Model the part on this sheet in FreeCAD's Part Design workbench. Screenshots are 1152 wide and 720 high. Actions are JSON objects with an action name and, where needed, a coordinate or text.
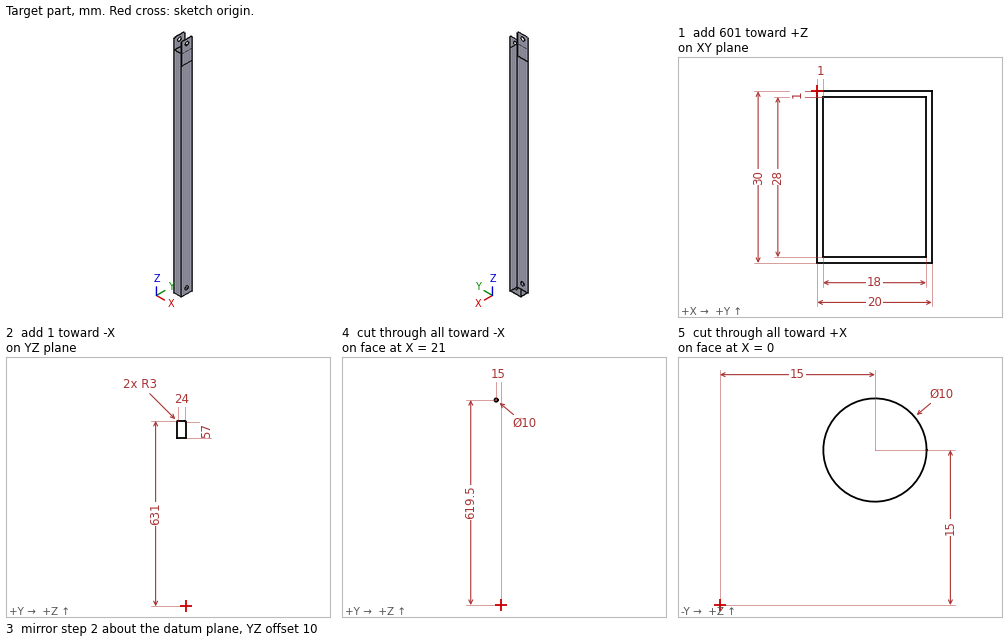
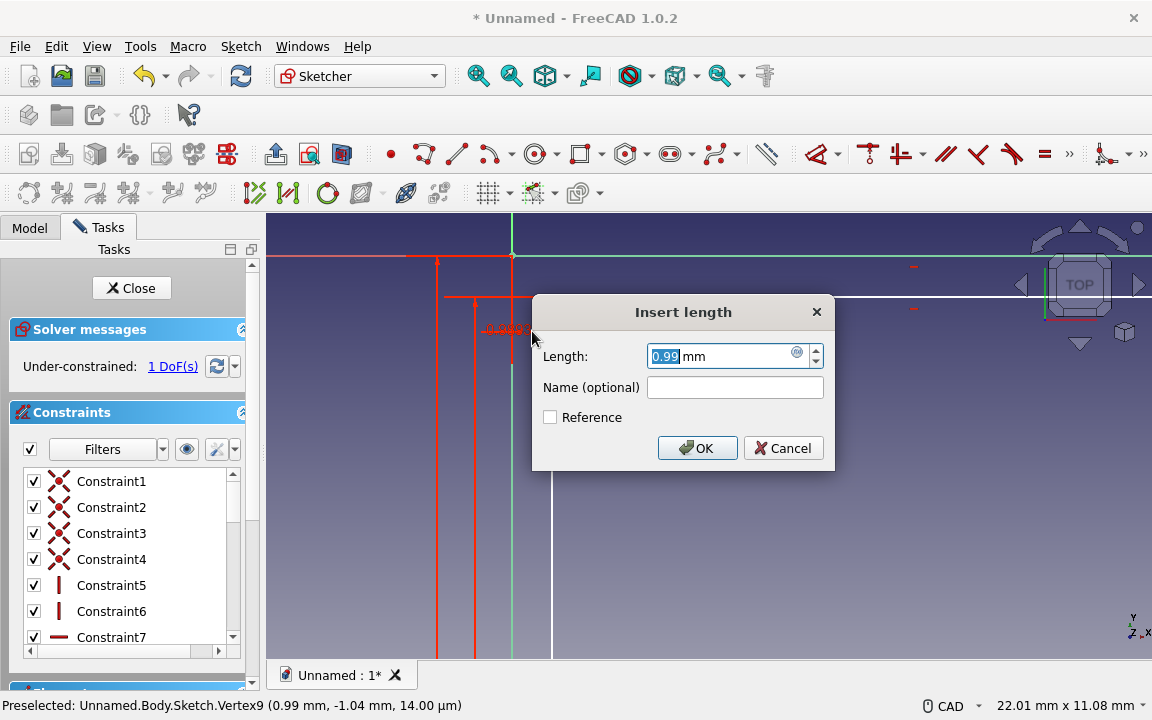
{"action": "type", "text": "1"}
{"action": "key", "text": "Return"}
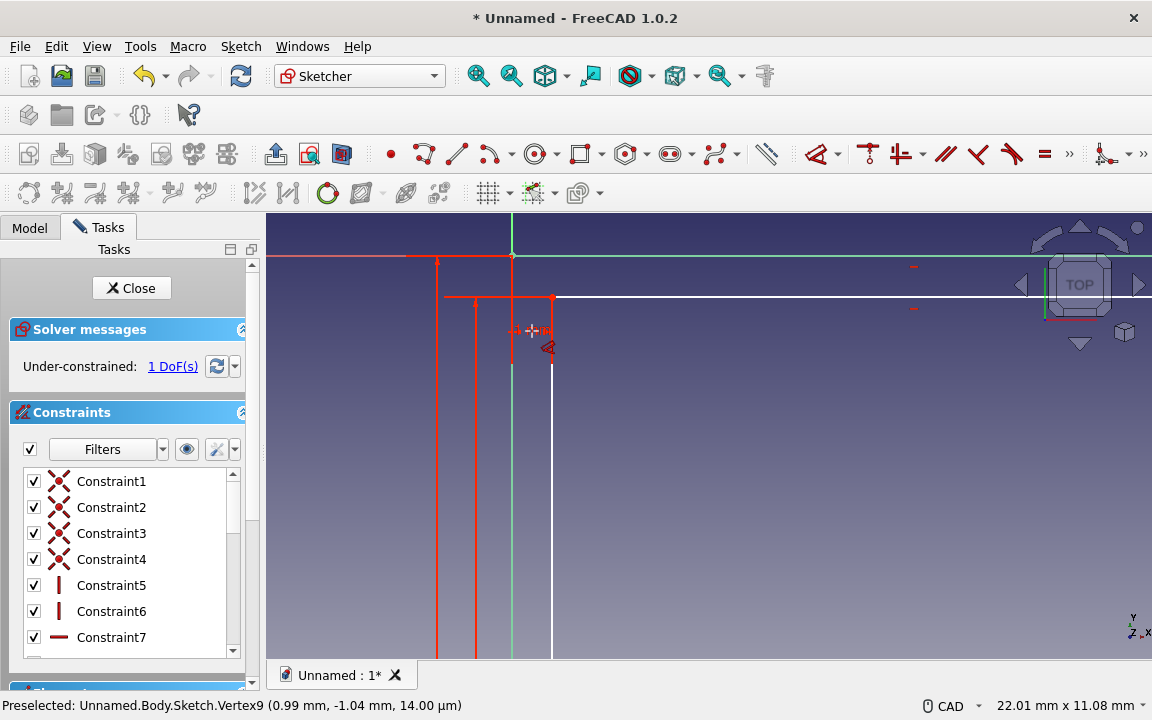
{"action": "left_click", "coordinate": [552, 297]}
{"action": "left_click", "coordinate": [478, 276]}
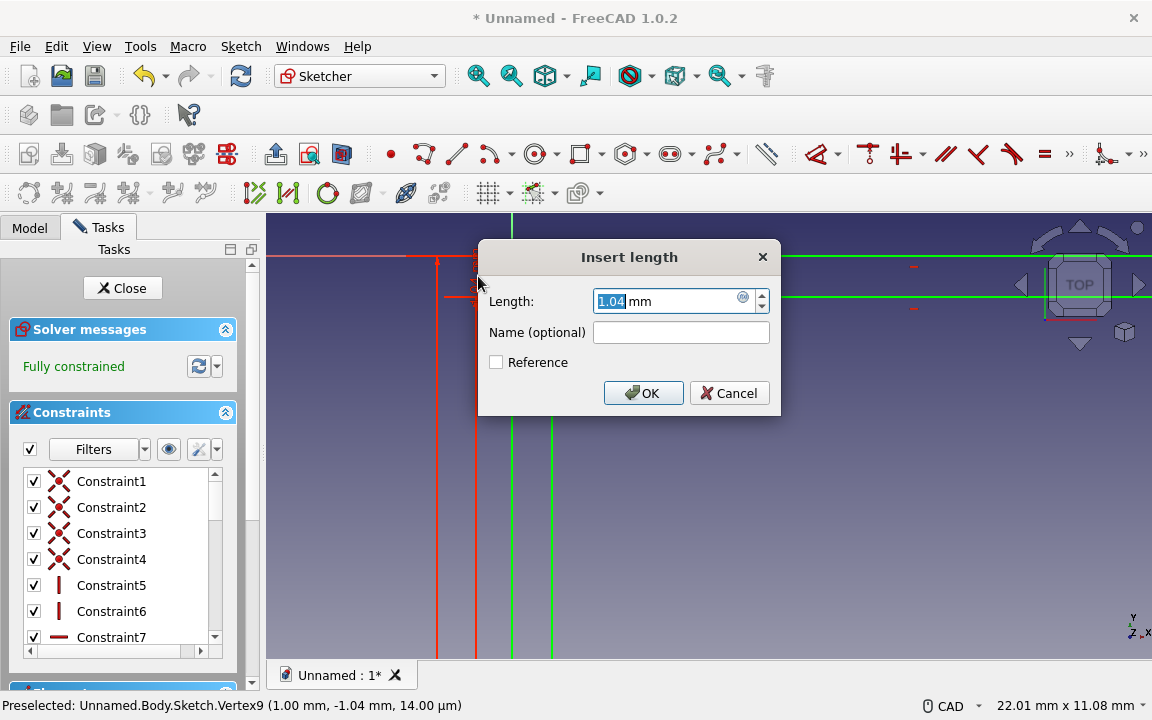
{"action": "type", "text": "1"}
{"action": "key", "text": "Return"}
{"action": "key", "text": "Escape"}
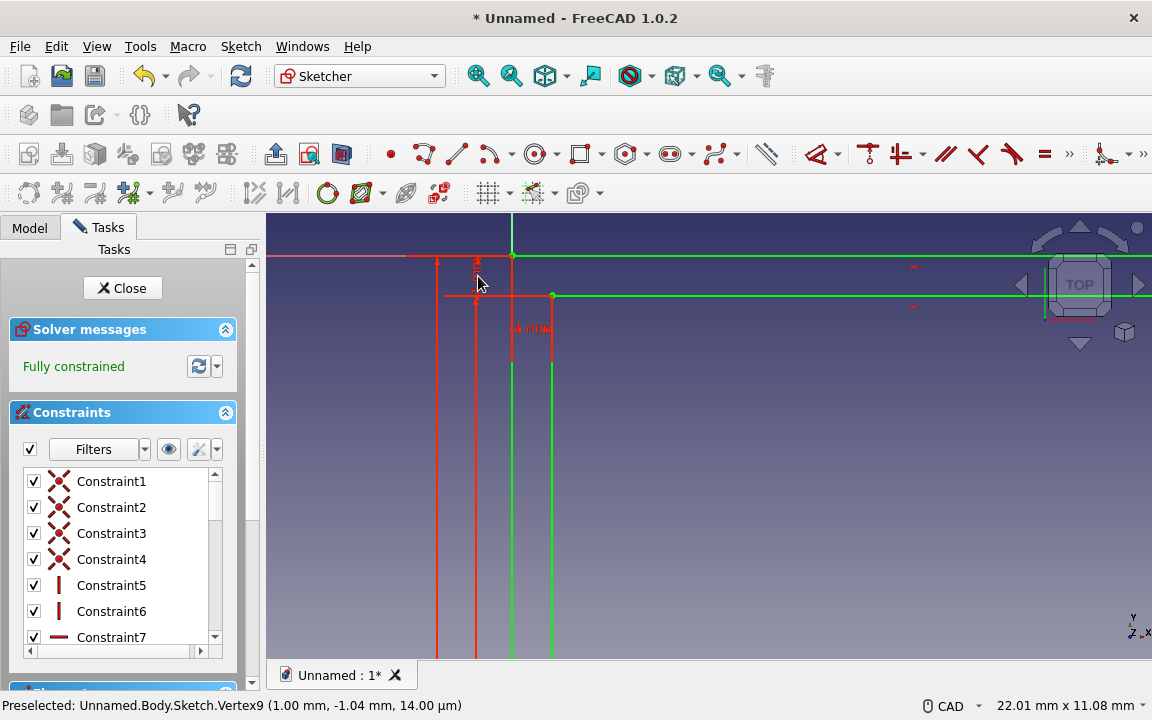
{"action": "left_click", "coordinate": [123, 288]}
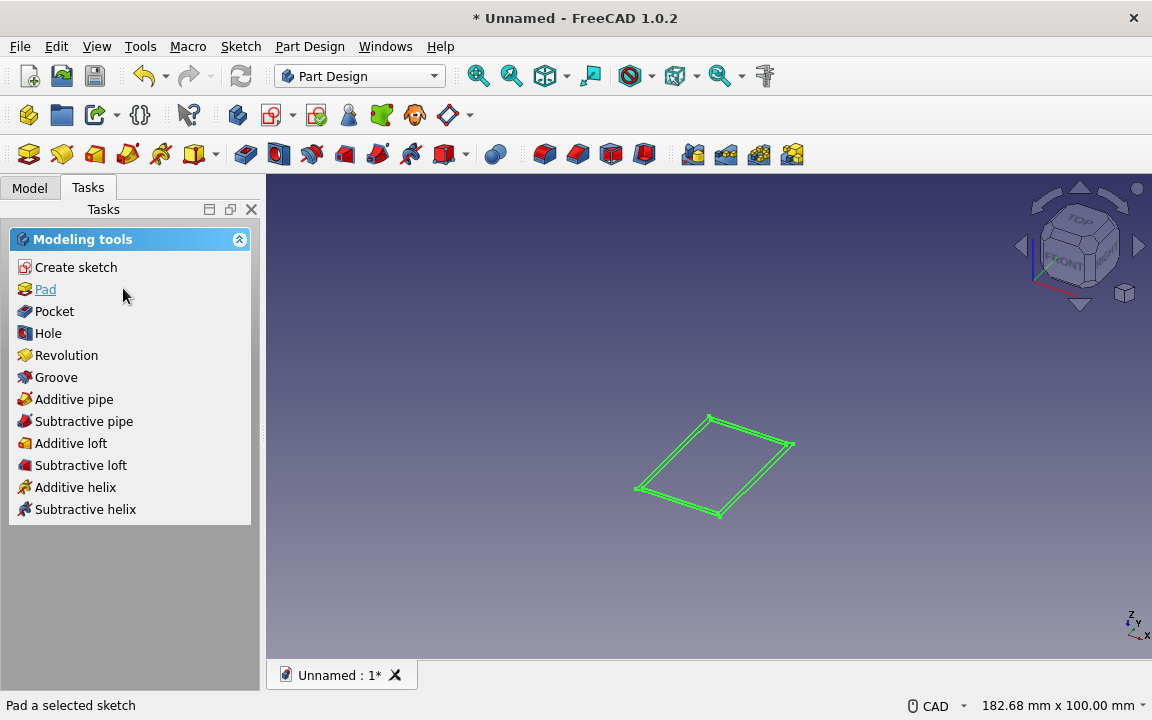
{"action": "left_click", "coordinate": [29, 154]}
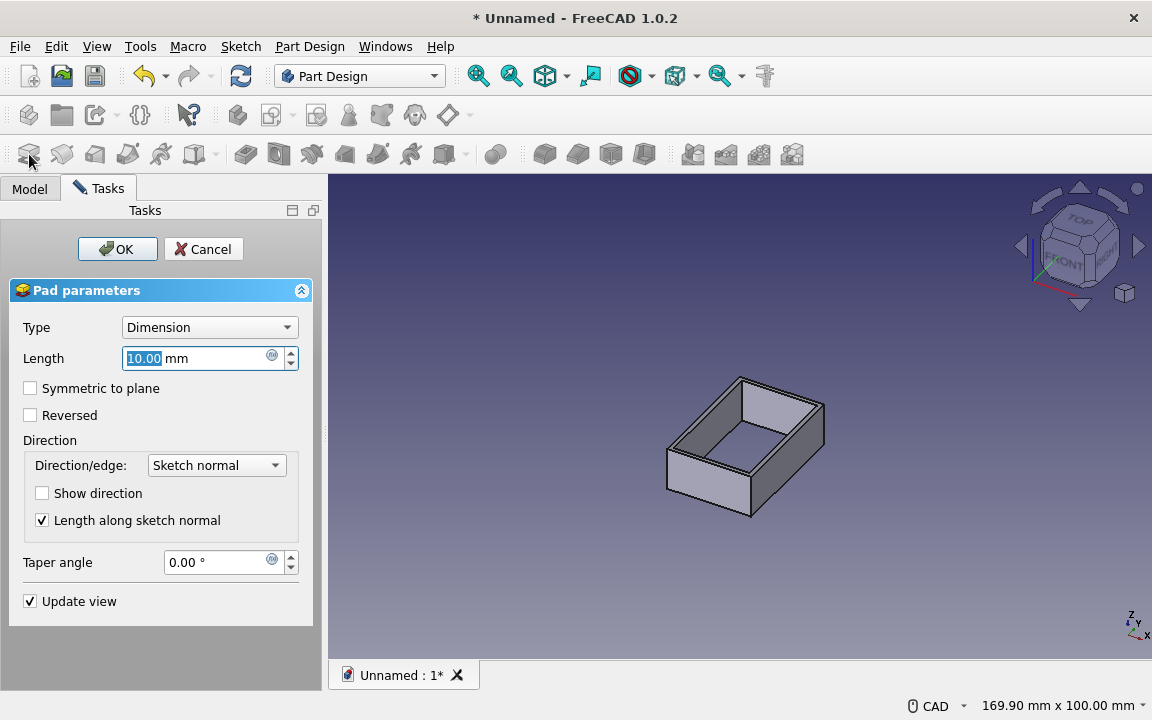
{"action": "type", "text": "601"}
{"action": "key", "text": "Tab"}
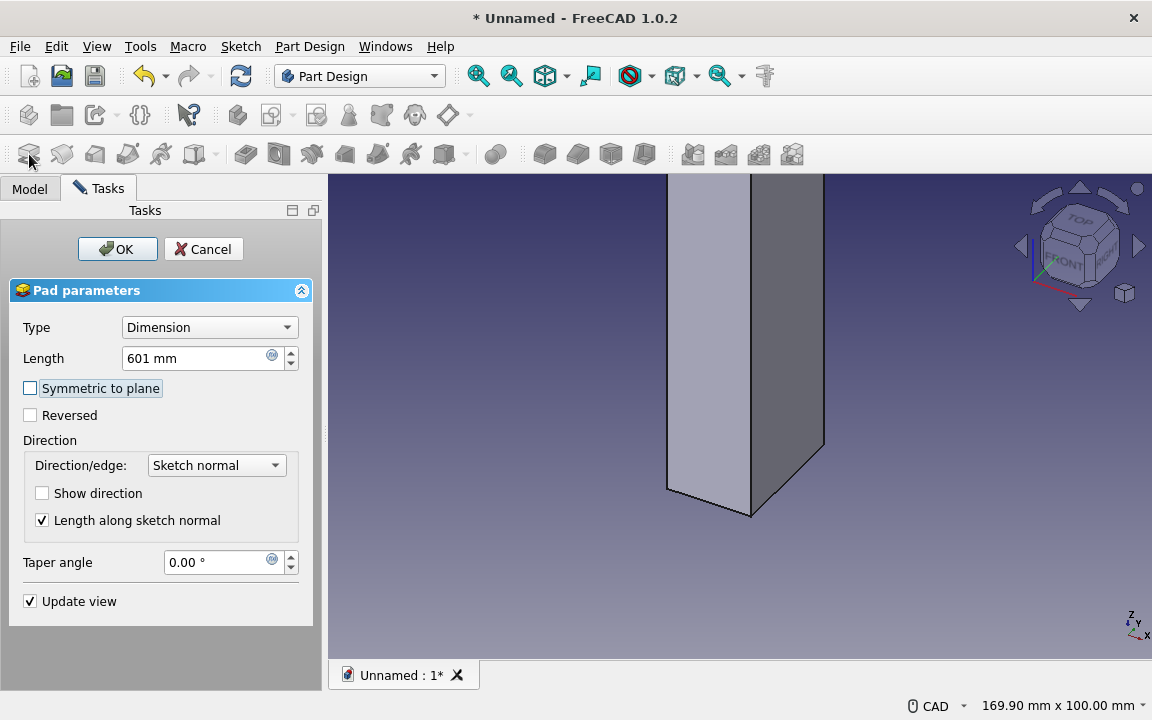
{"action": "left_click", "coordinate": [118, 249]}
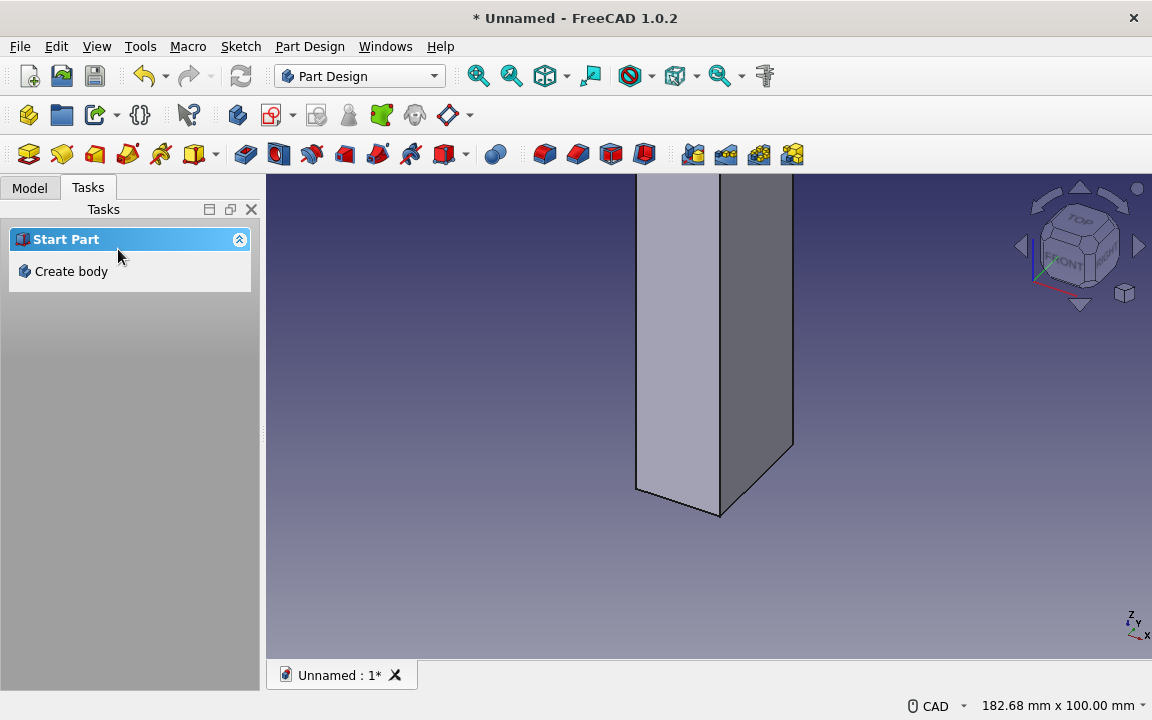
{"action": "key", "text": "v f"}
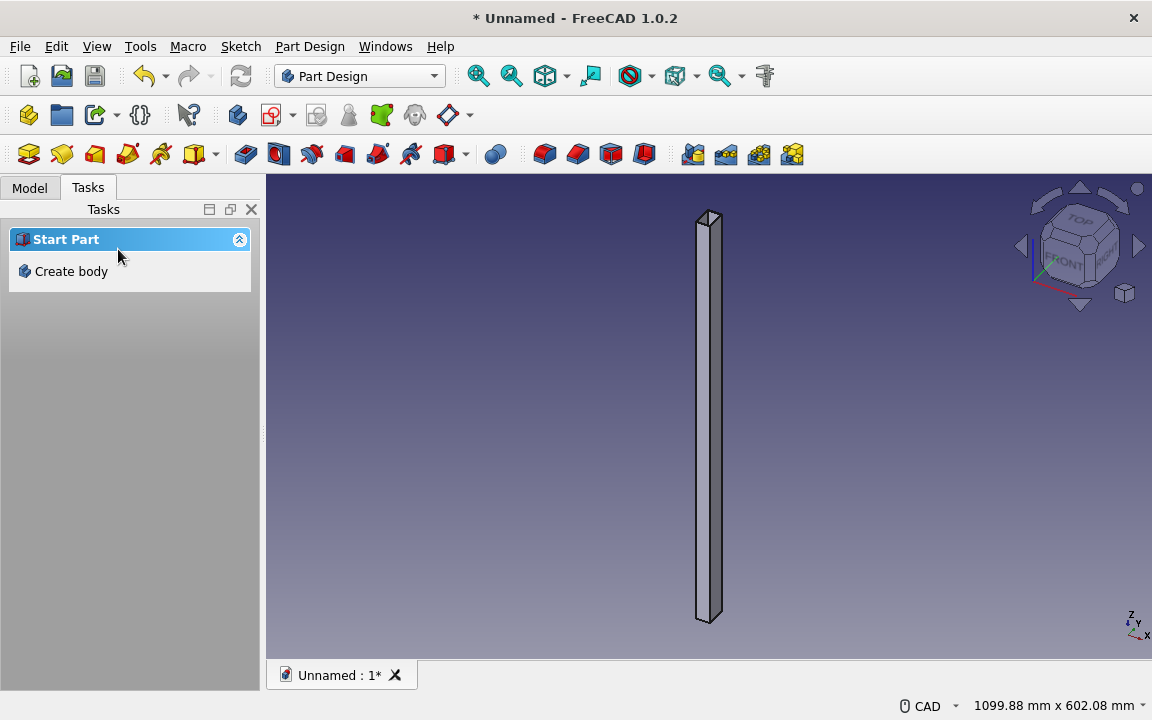
{"action": "left_click", "coordinate": [270, 116]}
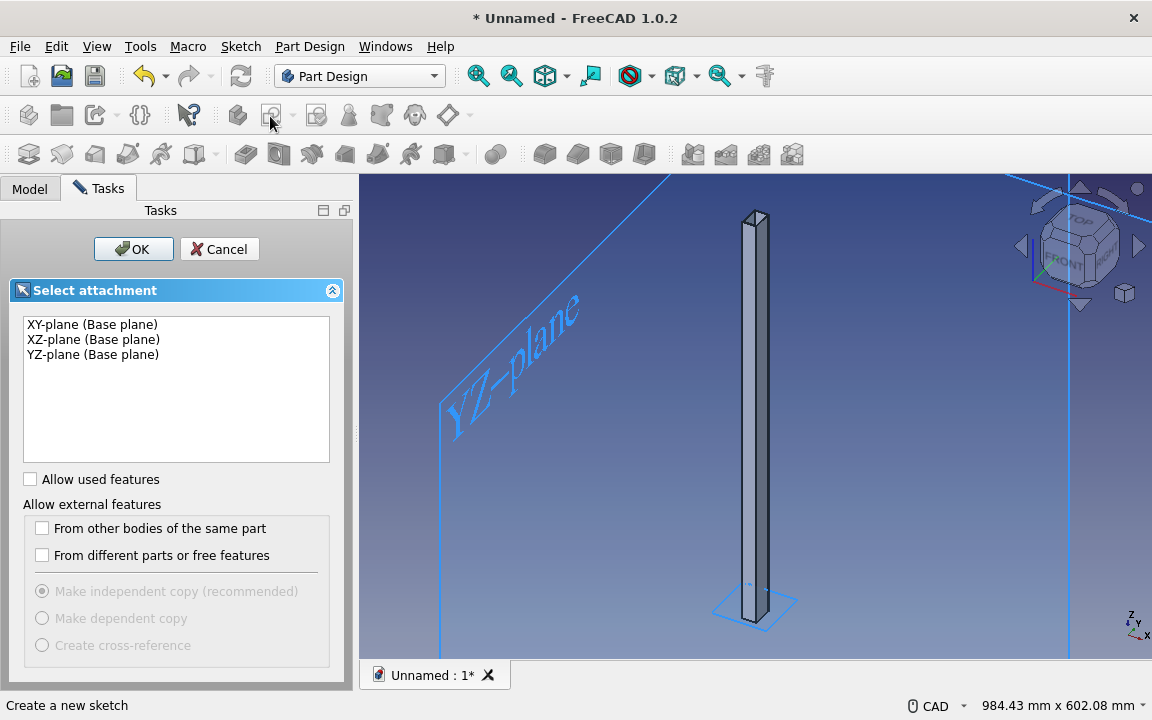
{"action": "left_click", "coordinate": [84, 354]}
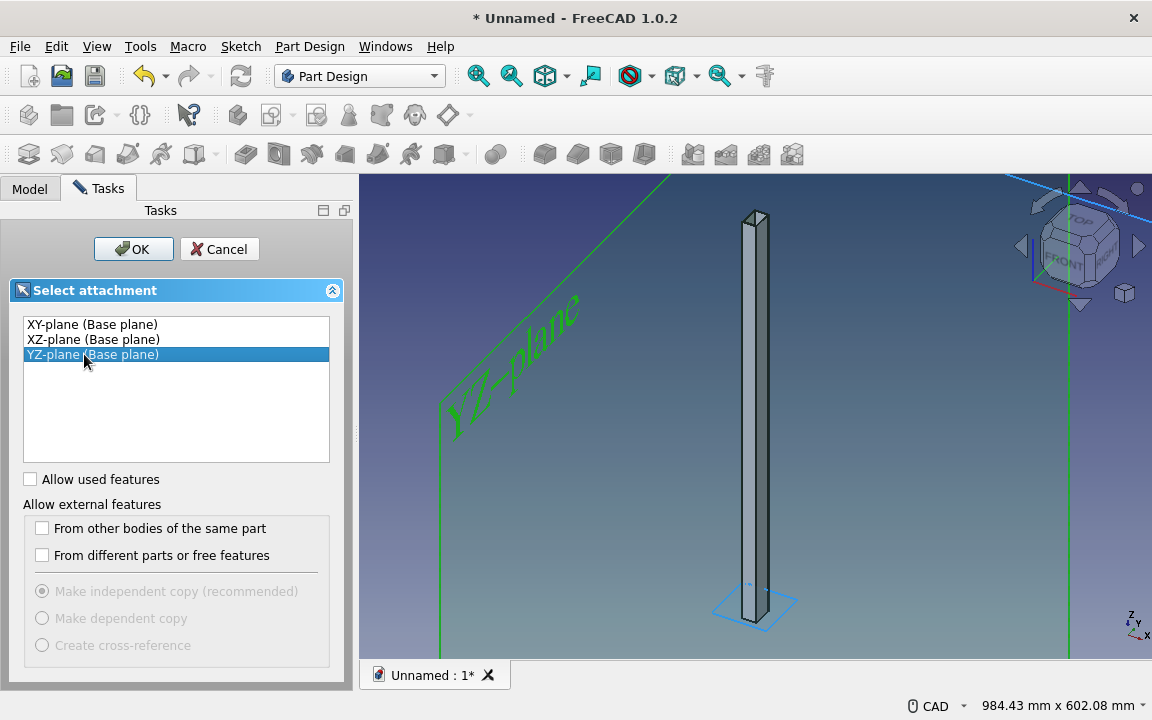
{"action": "left_click", "coordinate": [134, 249]}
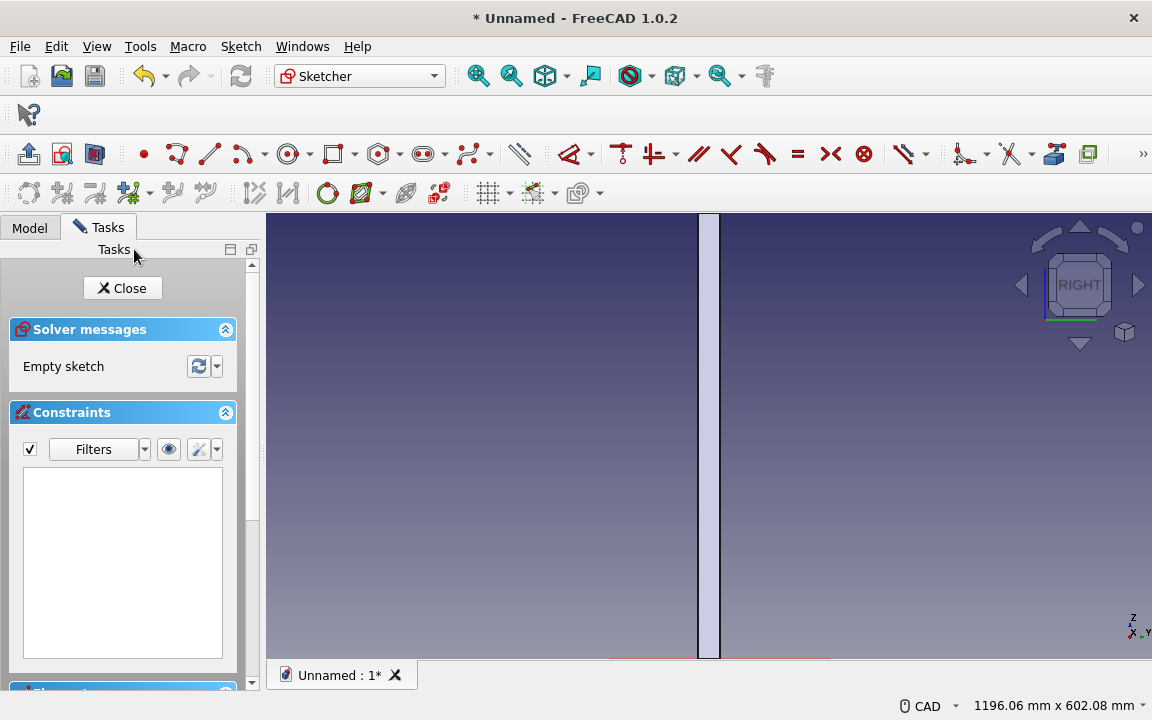
{"action": "key", "text": "q s"}